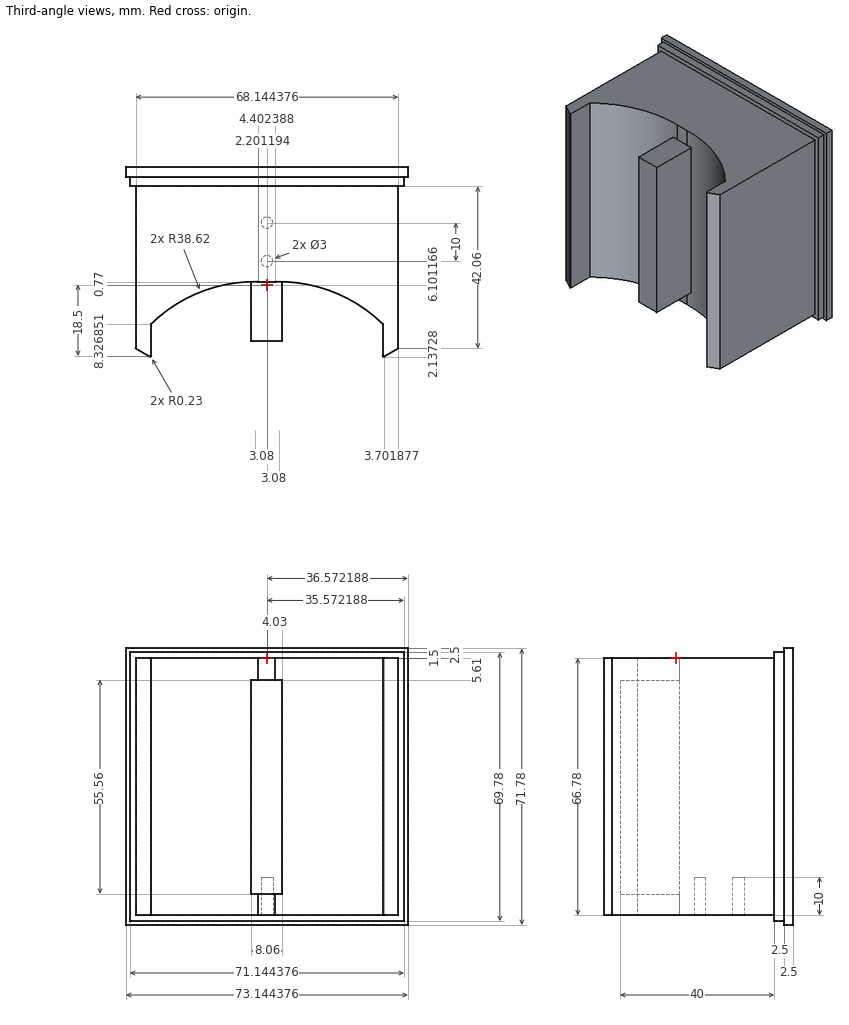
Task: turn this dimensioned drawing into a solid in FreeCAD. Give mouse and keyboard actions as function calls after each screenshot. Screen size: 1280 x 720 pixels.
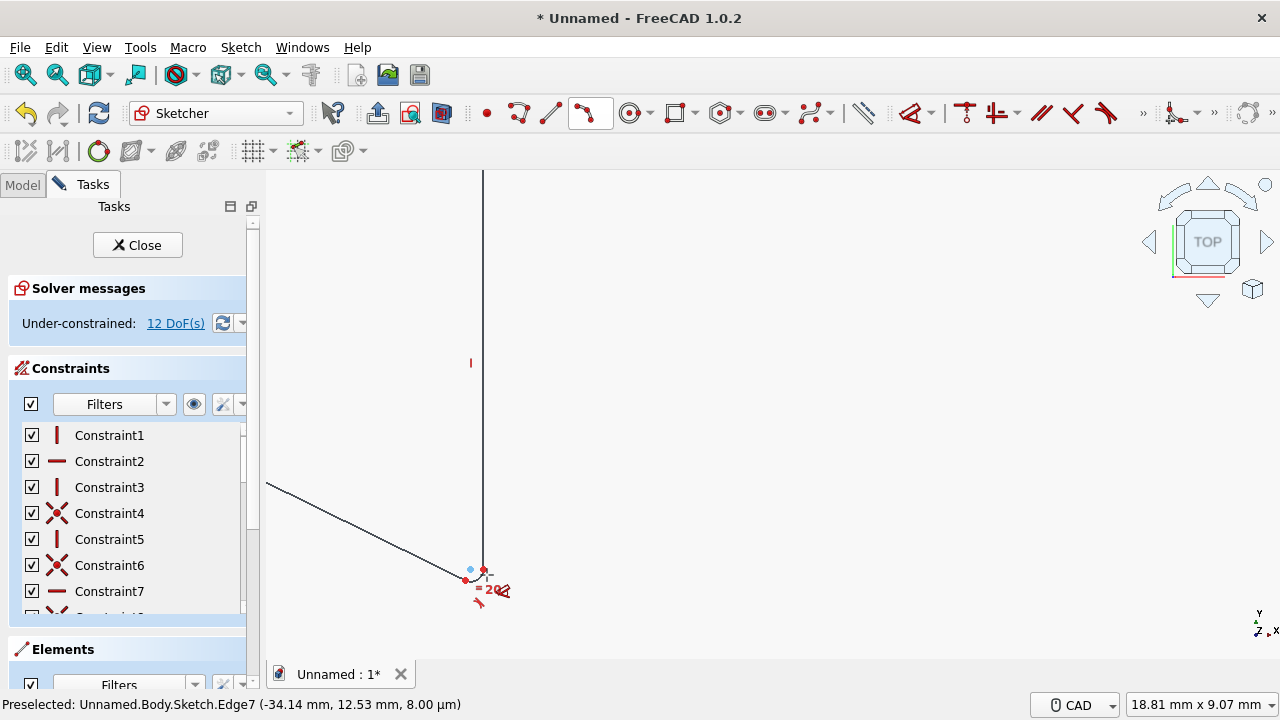
click(483, 569)
click(449, 384)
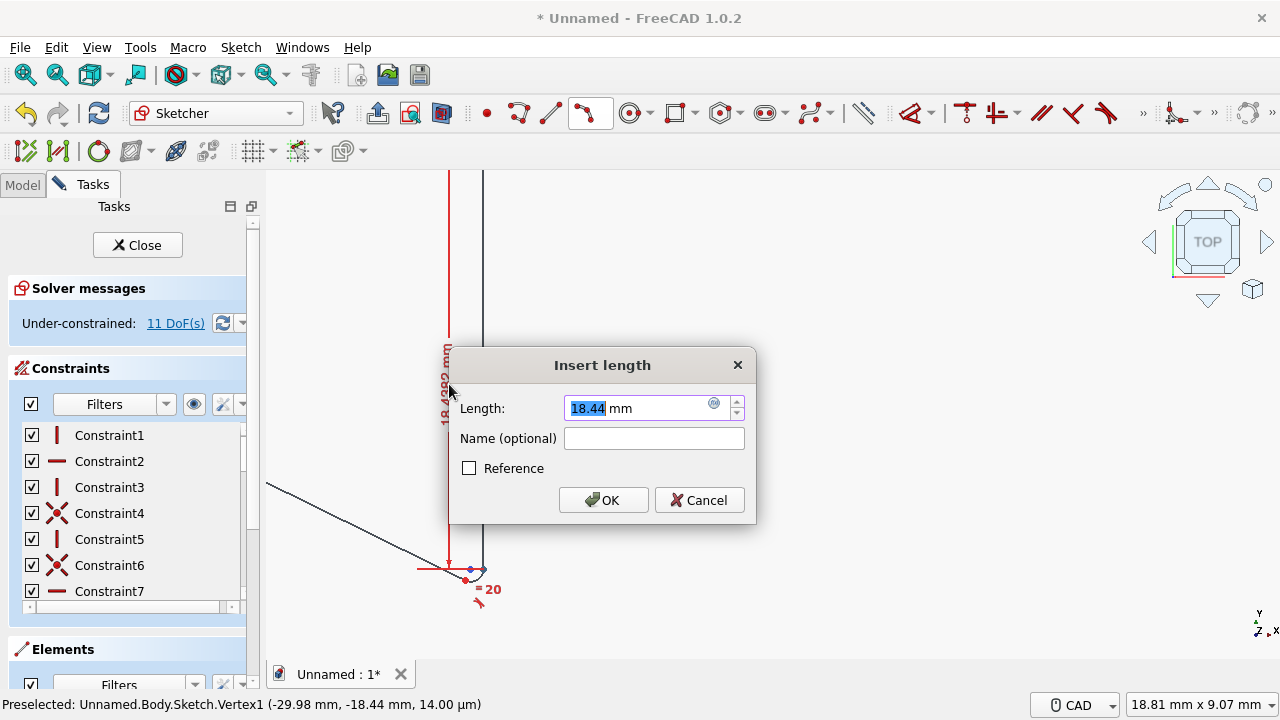
text(18.5)
key(Return)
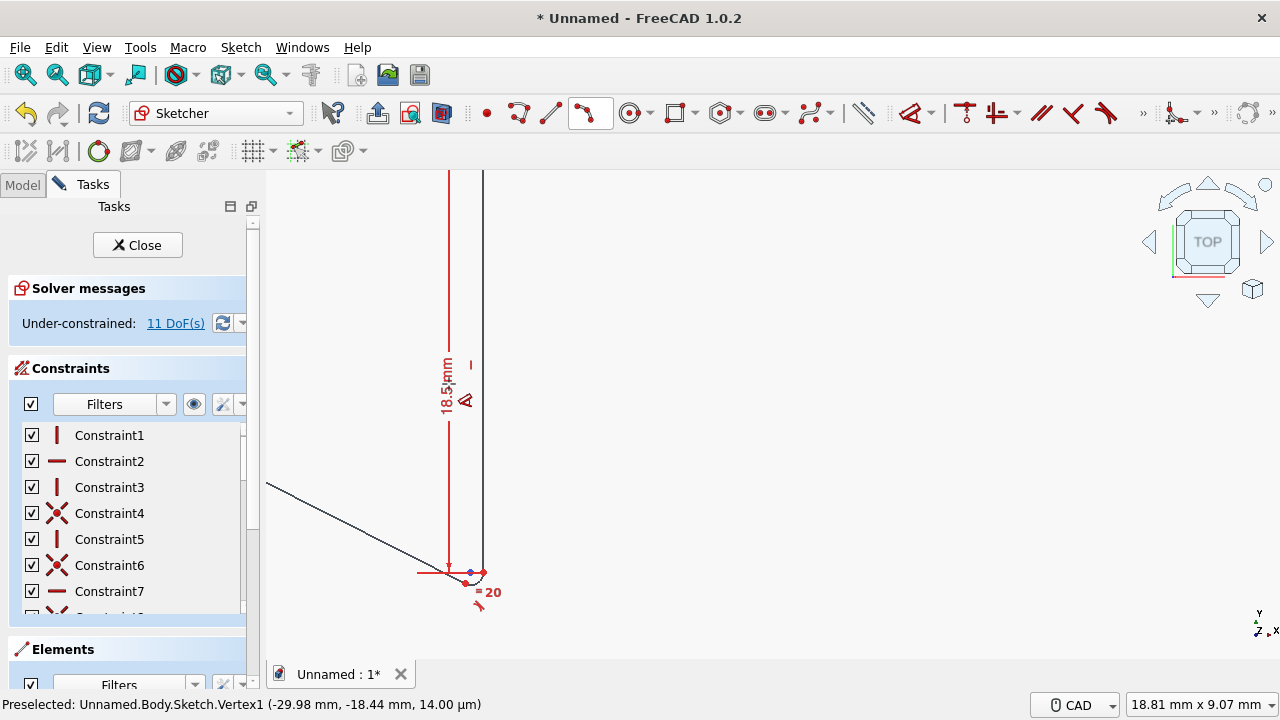
scroll(486, 575, down, 10)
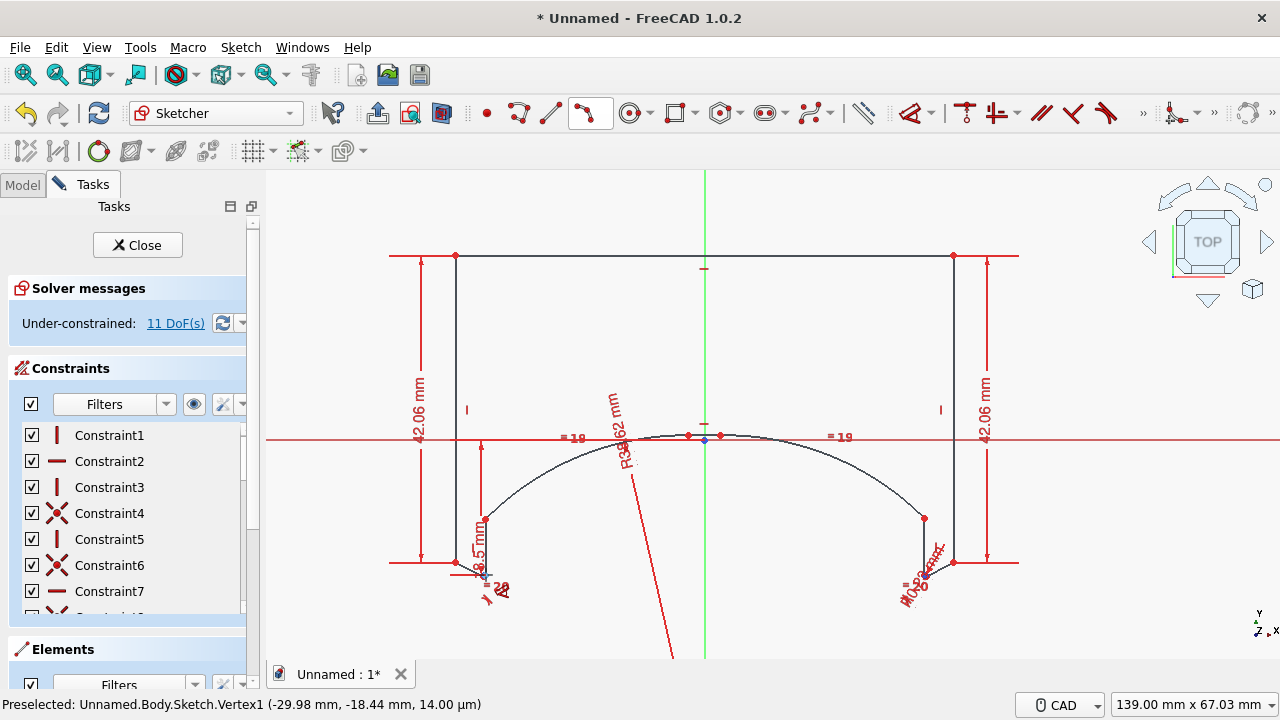
scroll(688, 435, up, 10)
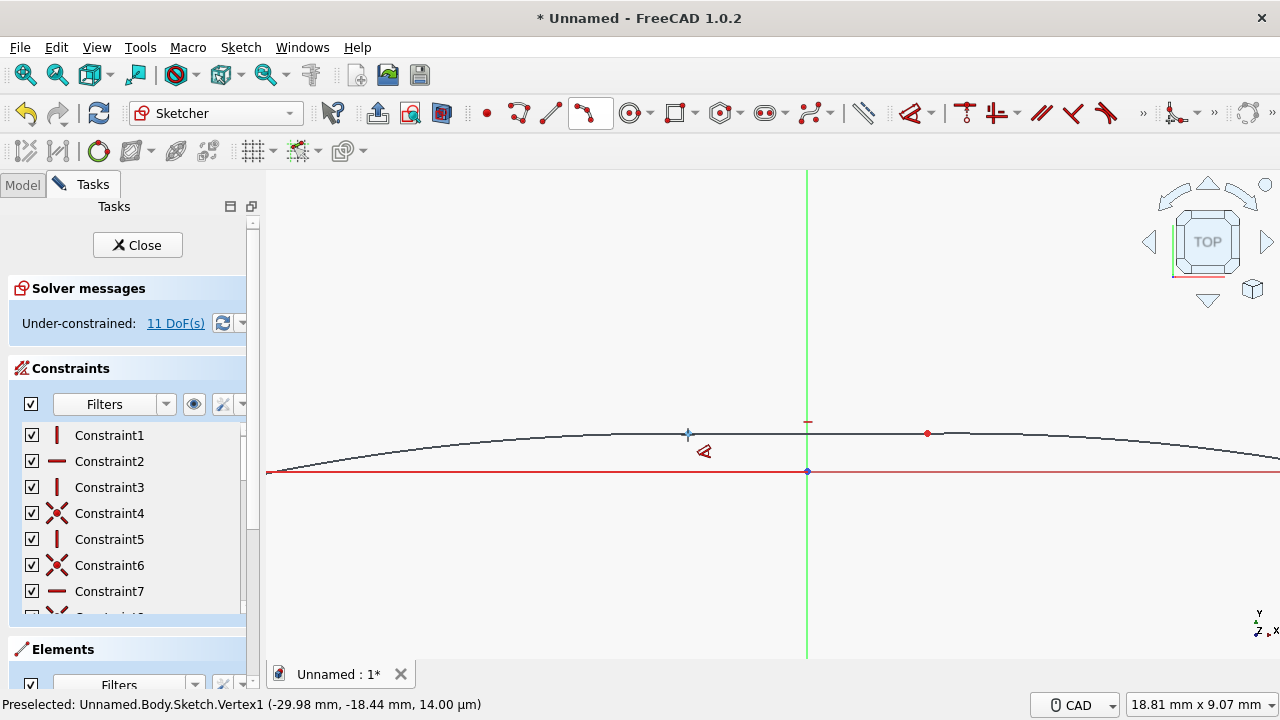
click(689, 434)
click(655, 453)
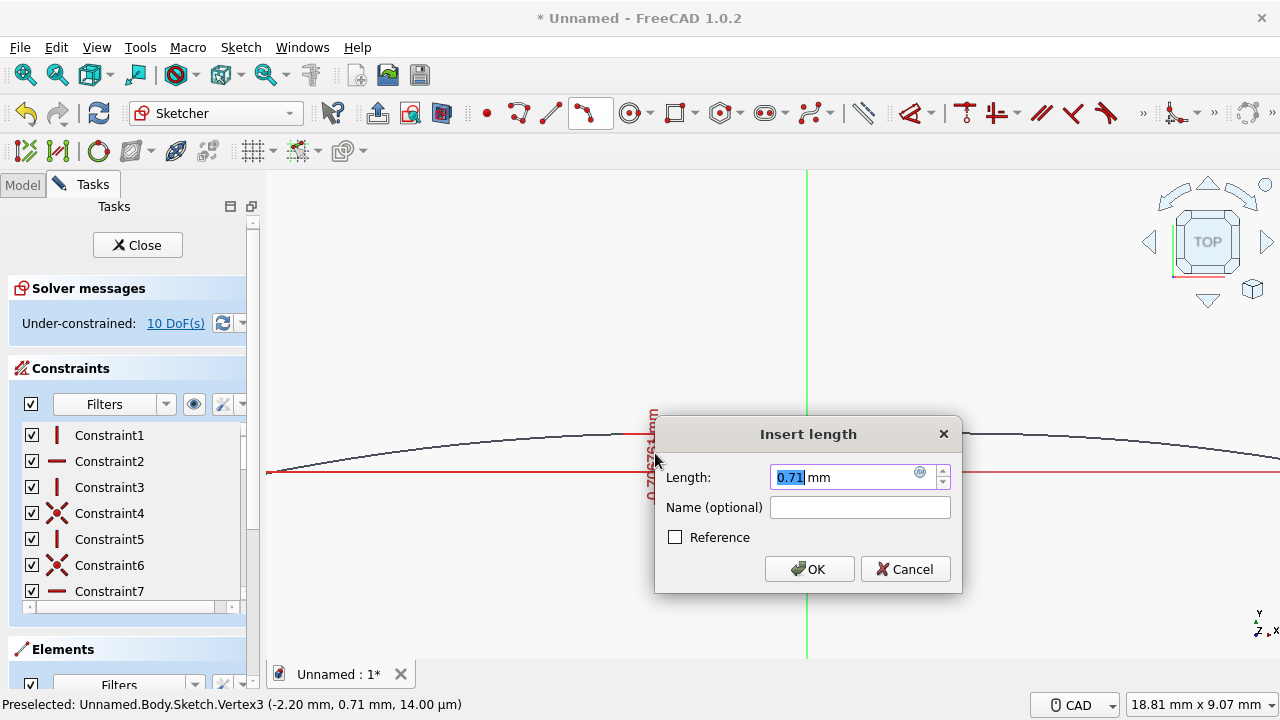
text(0.77)
key(Return)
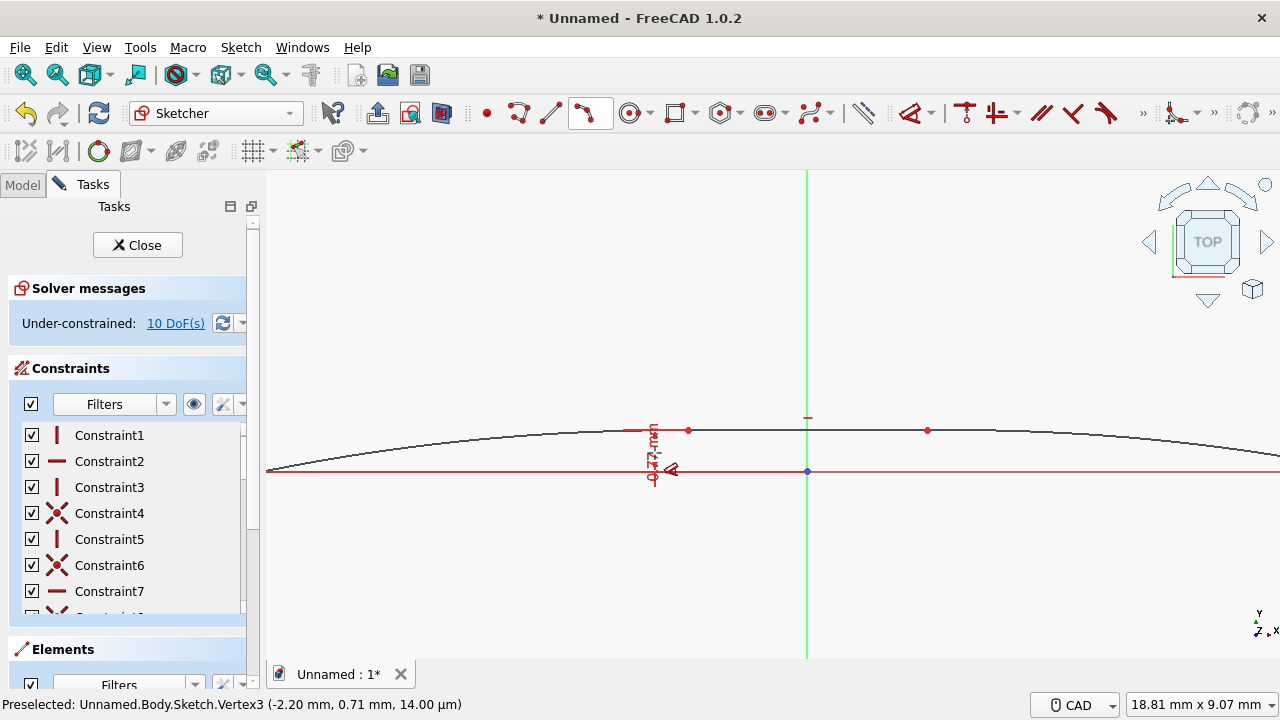
scroll(688, 434, down, 10)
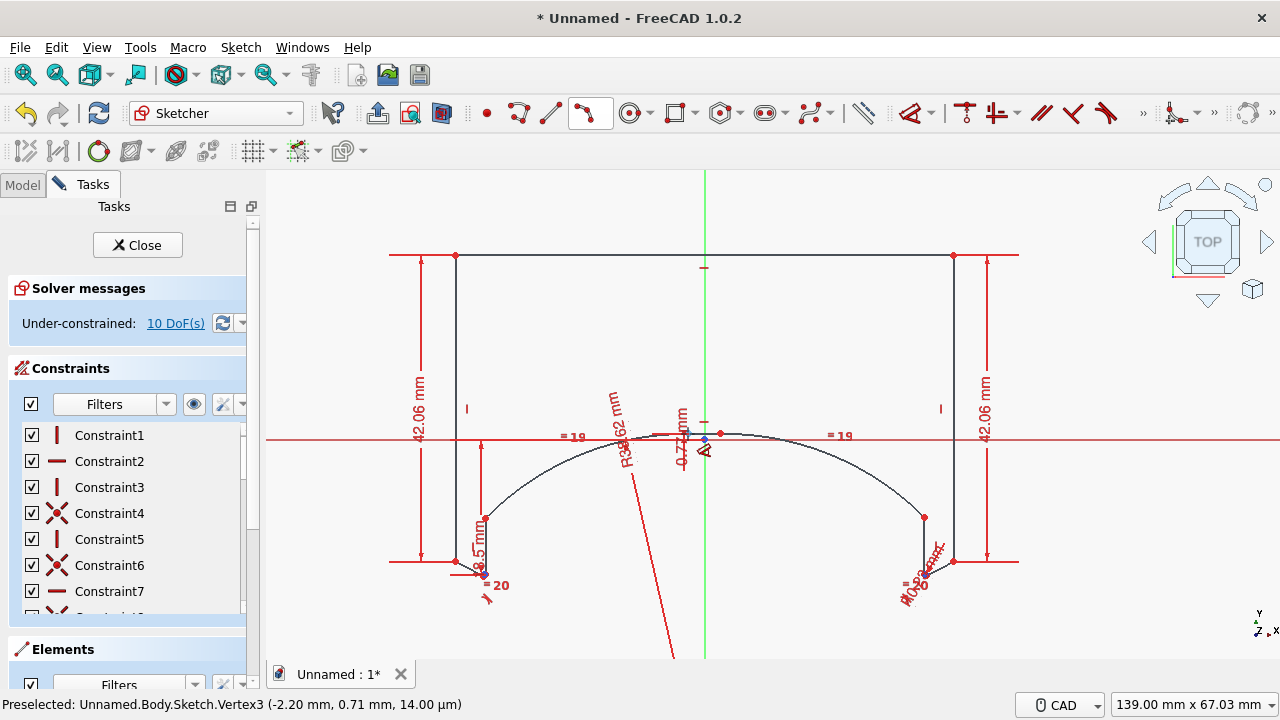
scroll(924, 574, up, 10)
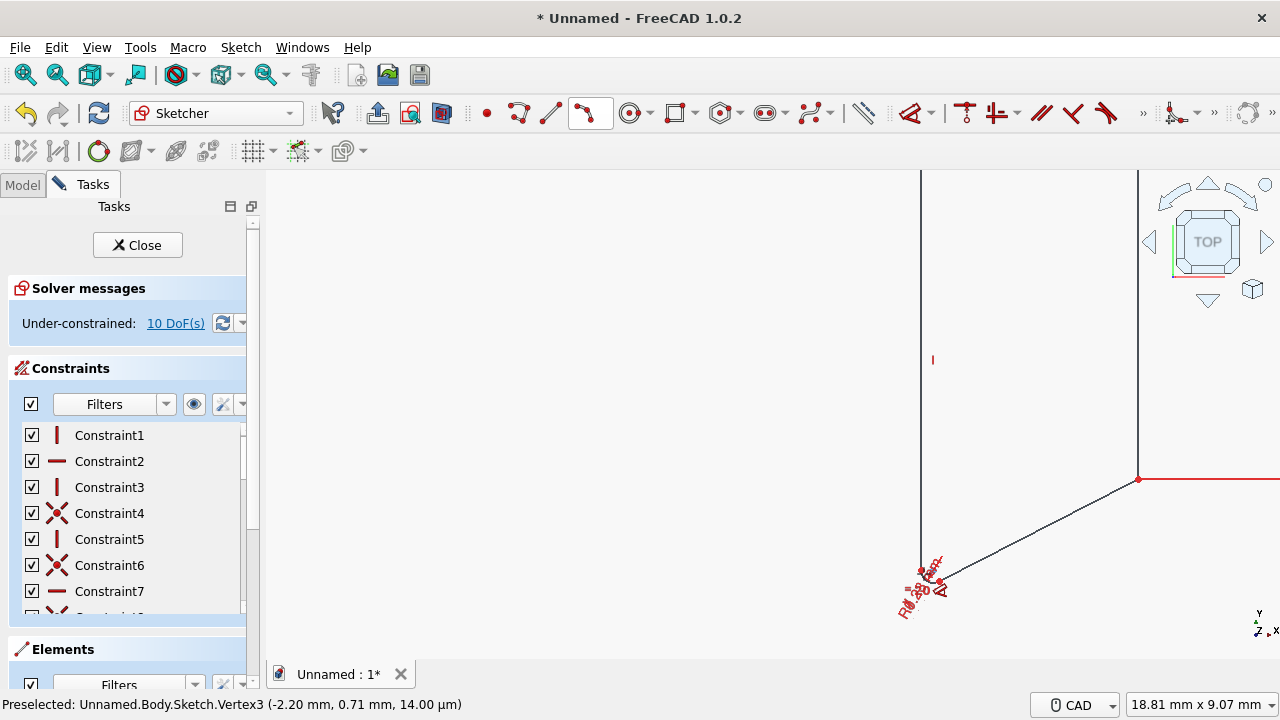
click(921, 570)
click(955, 384)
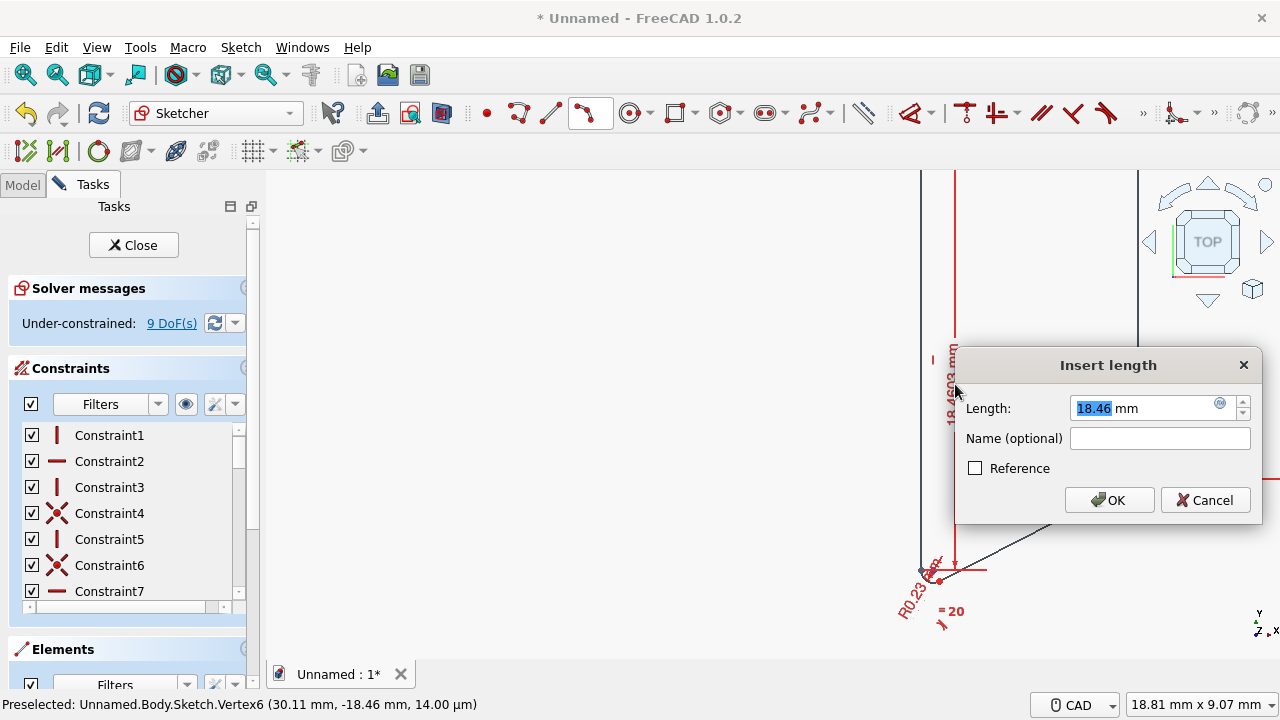
text(18.5)
key(Return)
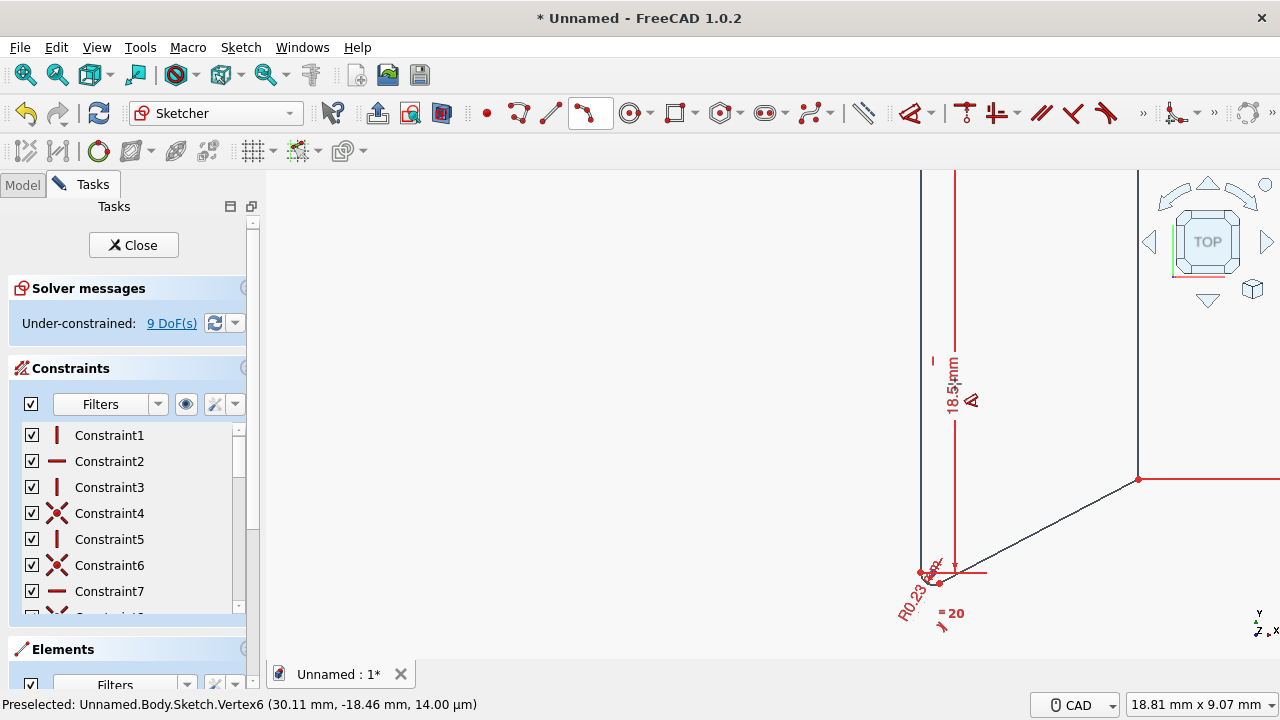
scroll(925, 575, down, 10)